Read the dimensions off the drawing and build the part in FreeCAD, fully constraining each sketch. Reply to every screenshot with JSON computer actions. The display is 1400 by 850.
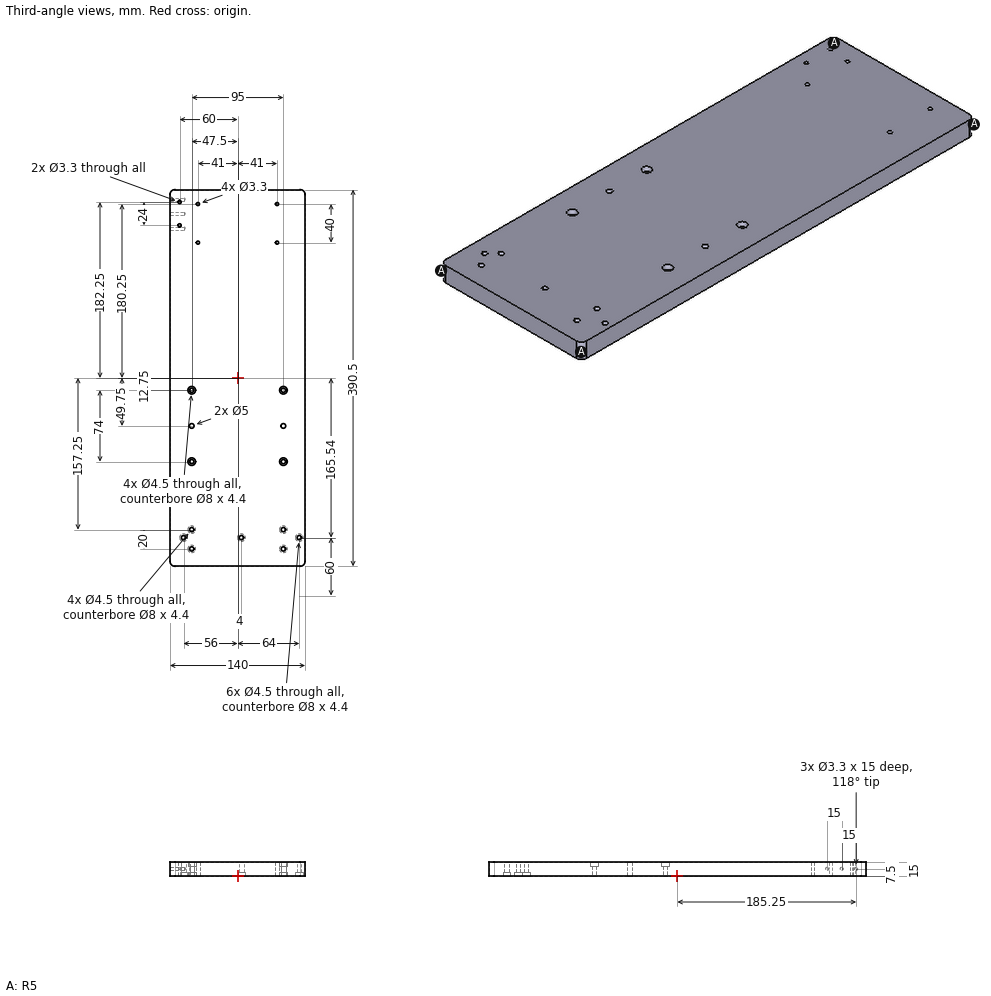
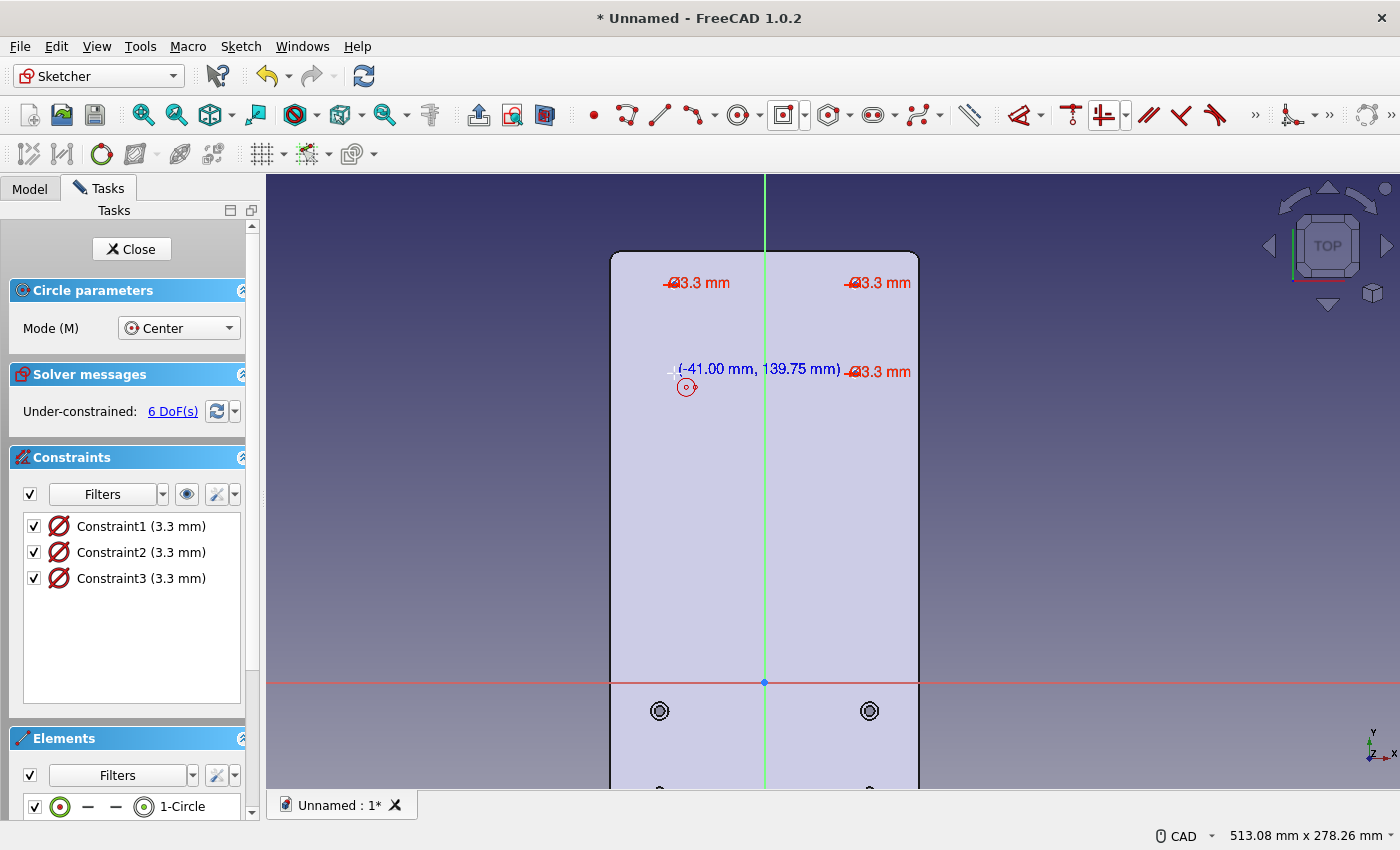
{"action": "left_click", "coordinate": [674, 373]}
{"action": "mouse_move", "coordinate": [677, 370]}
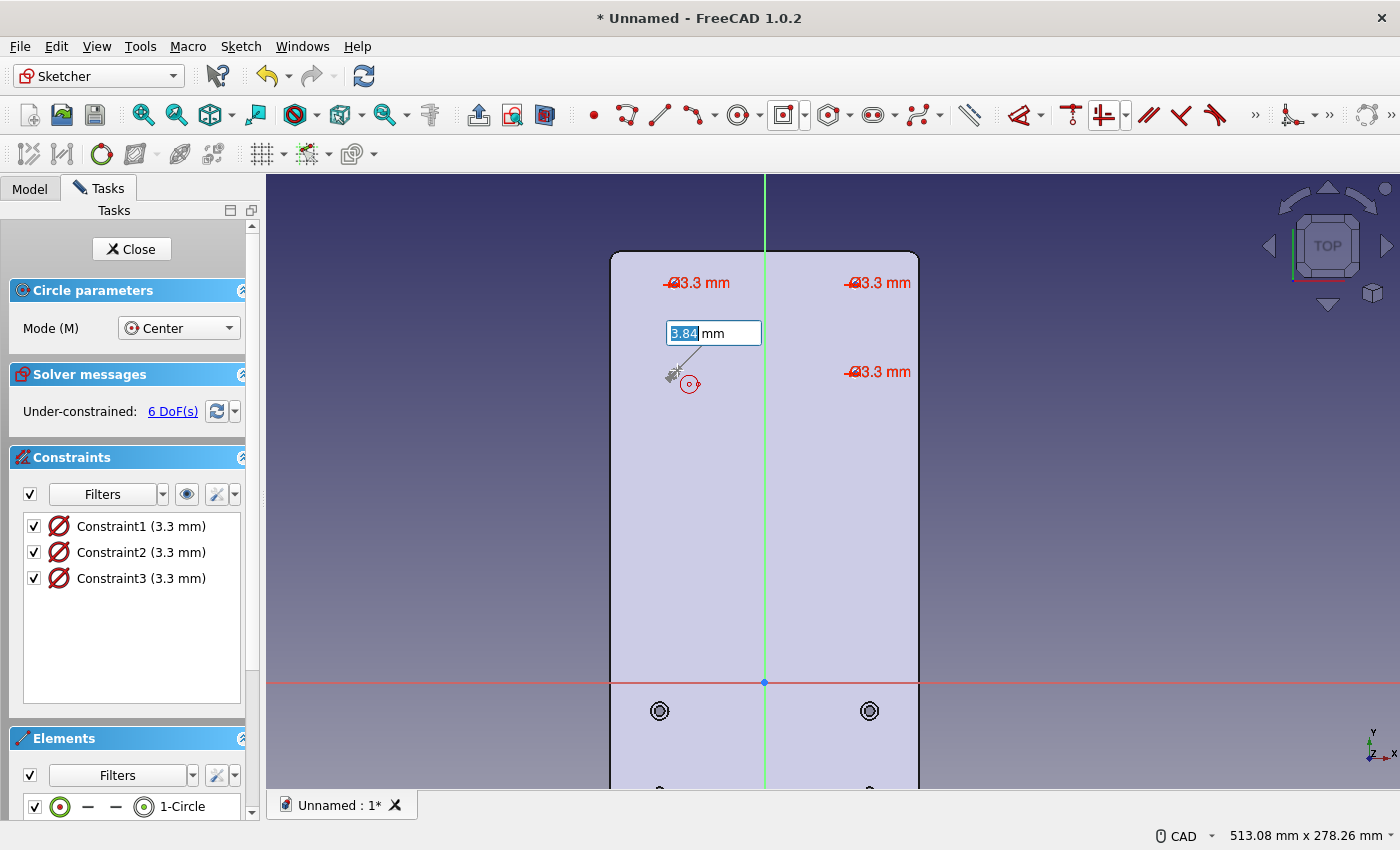
{"action": "type", "text": "3.3"}
{"action": "key", "text": "Return"}
{"action": "key", "text": "Escape"}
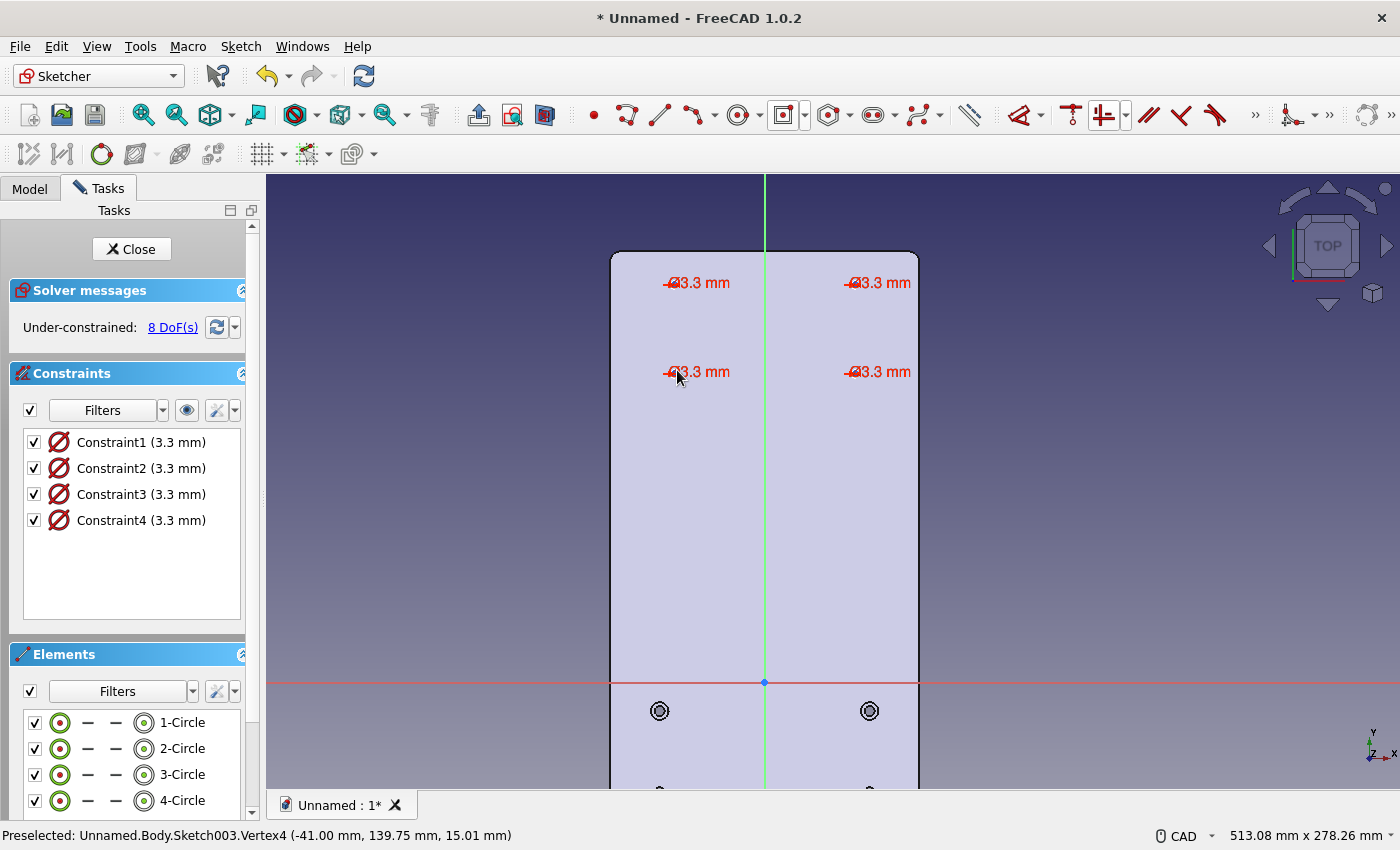
{"action": "left_click", "coordinate": [674, 285]}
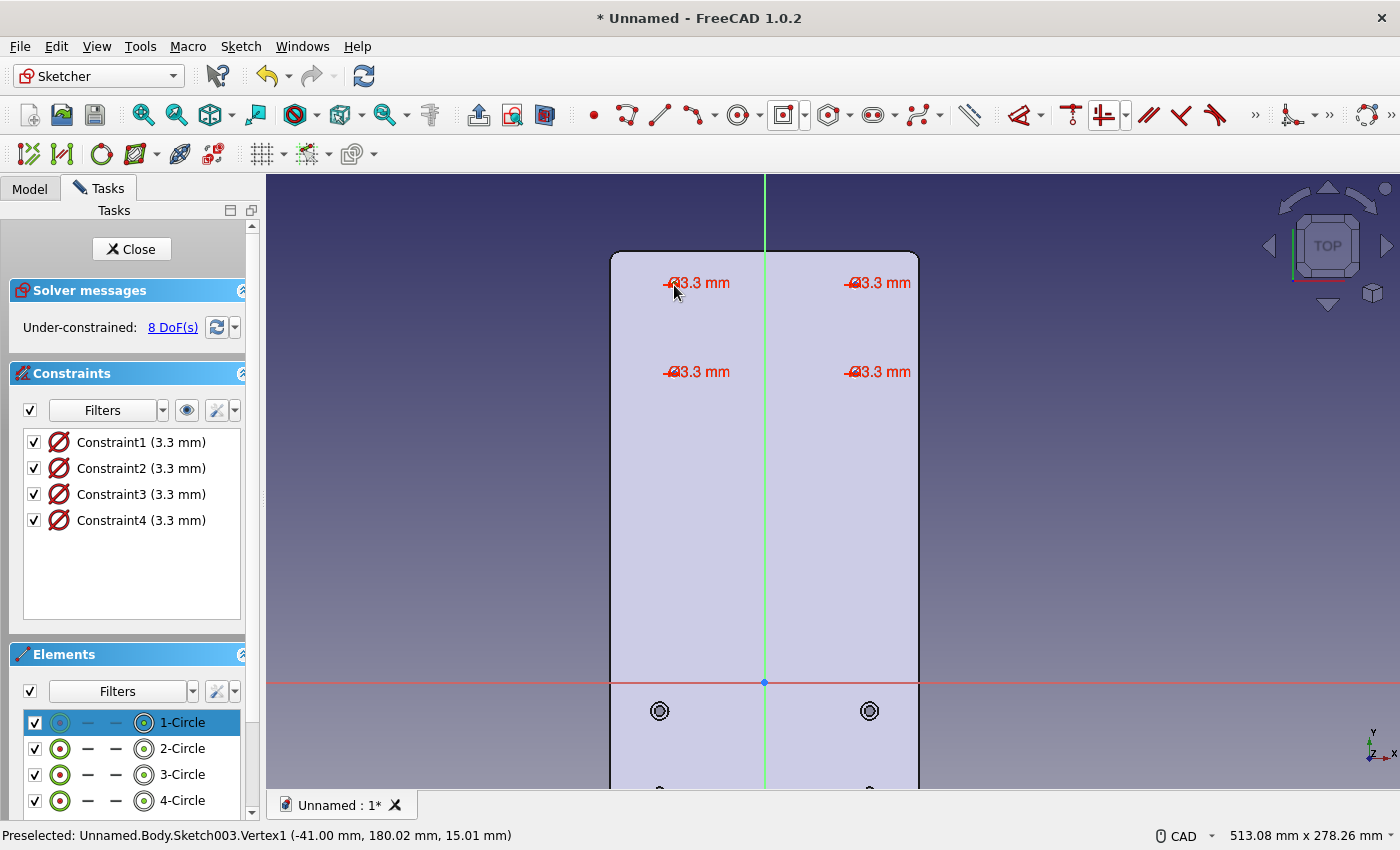
{"action": "left_click", "coordinate": [855, 285]}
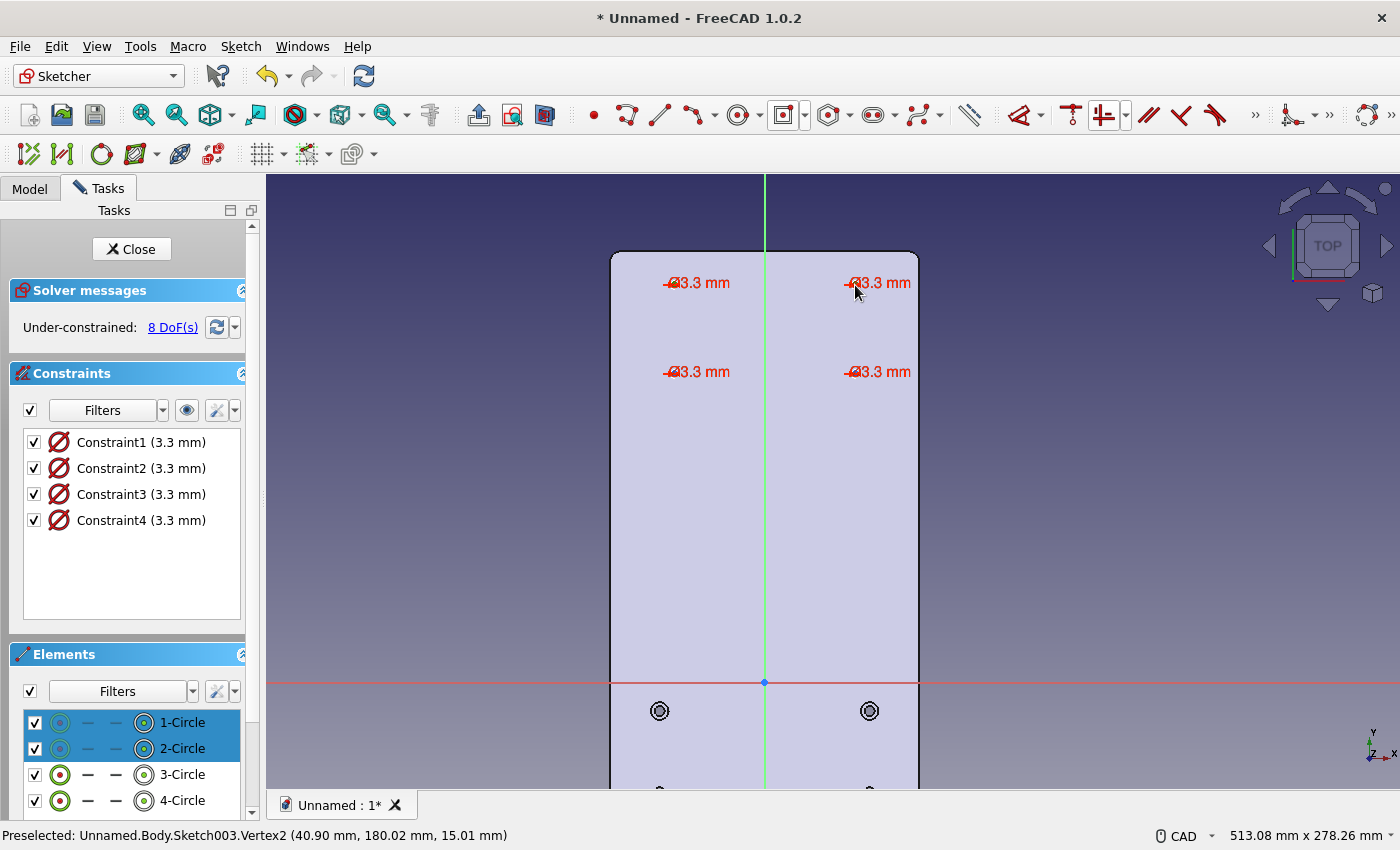
{"action": "key", "text": "h"}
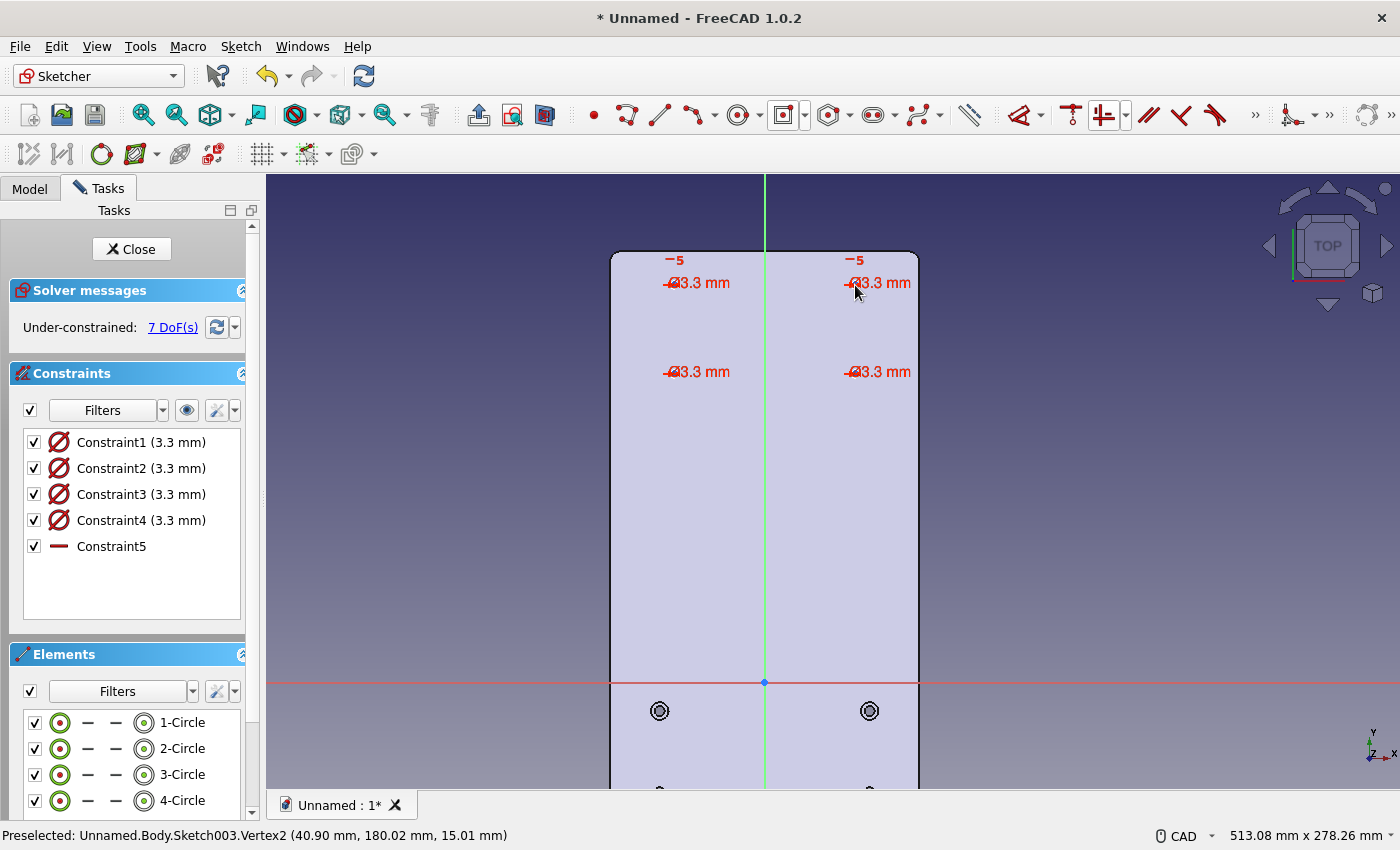
{"action": "left_click", "coordinate": [855, 285]}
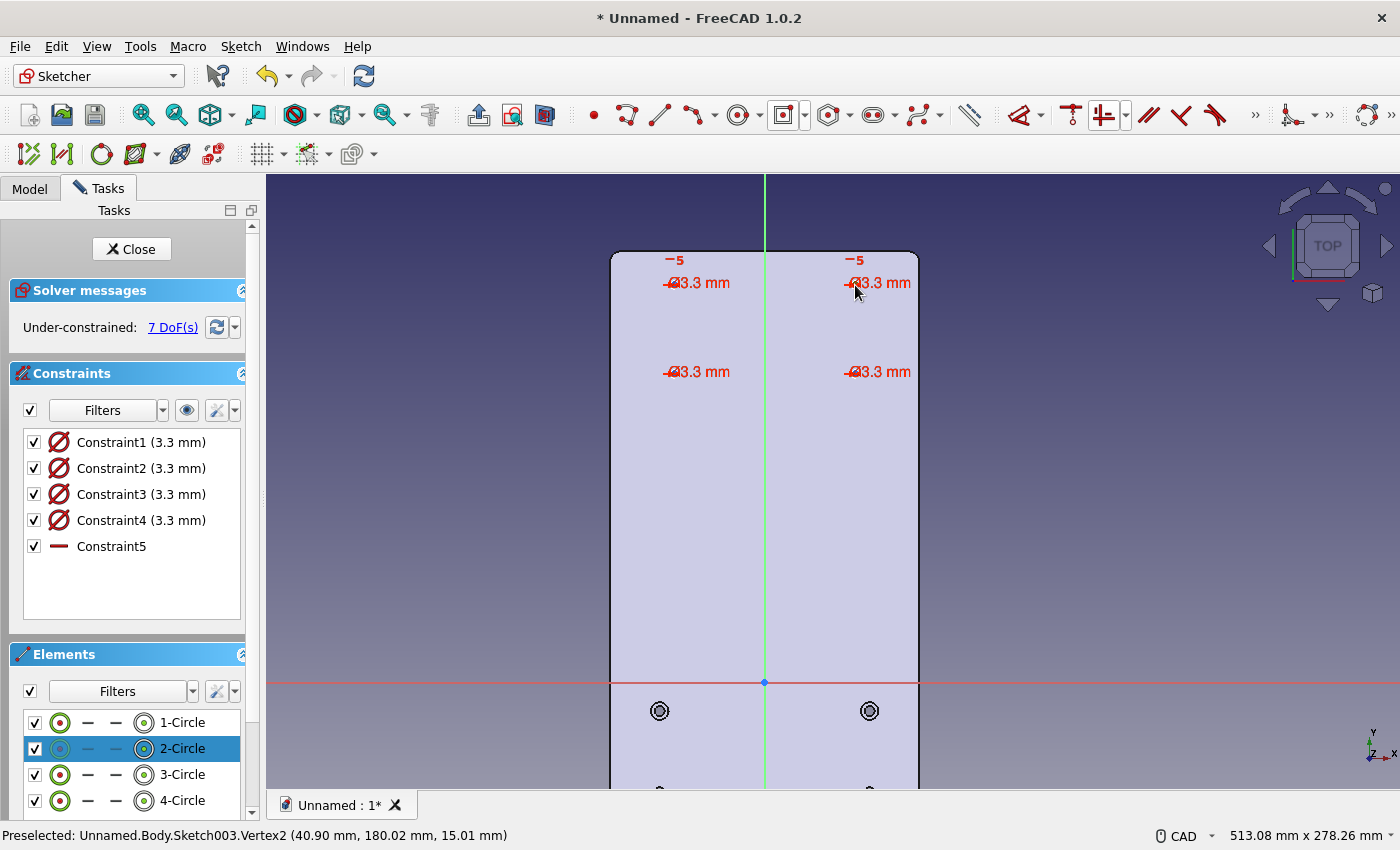
{"action": "left_click", "coordinate": [855, 374]}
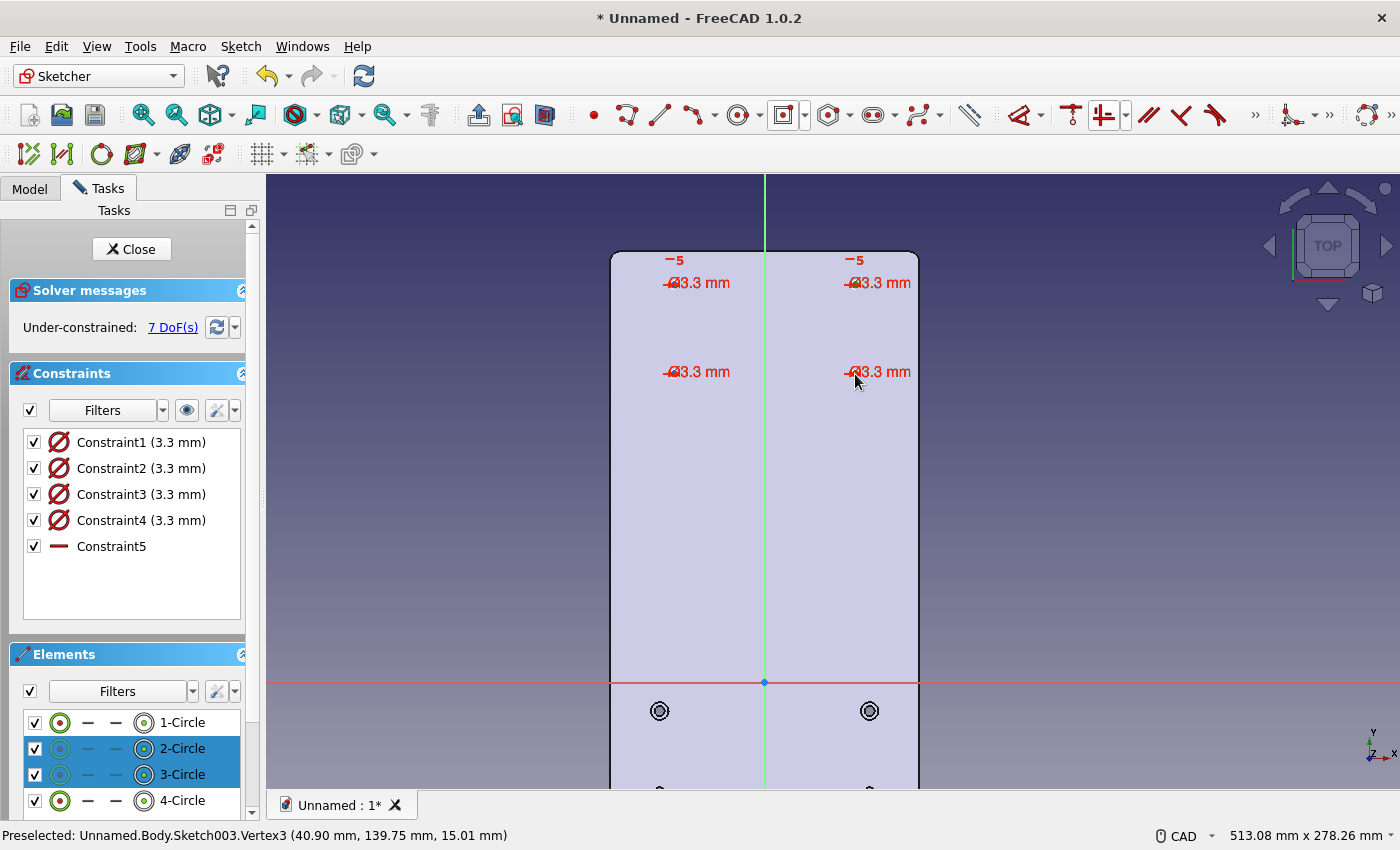
{"action": "left_click", "coordinate": [1126, 116]}